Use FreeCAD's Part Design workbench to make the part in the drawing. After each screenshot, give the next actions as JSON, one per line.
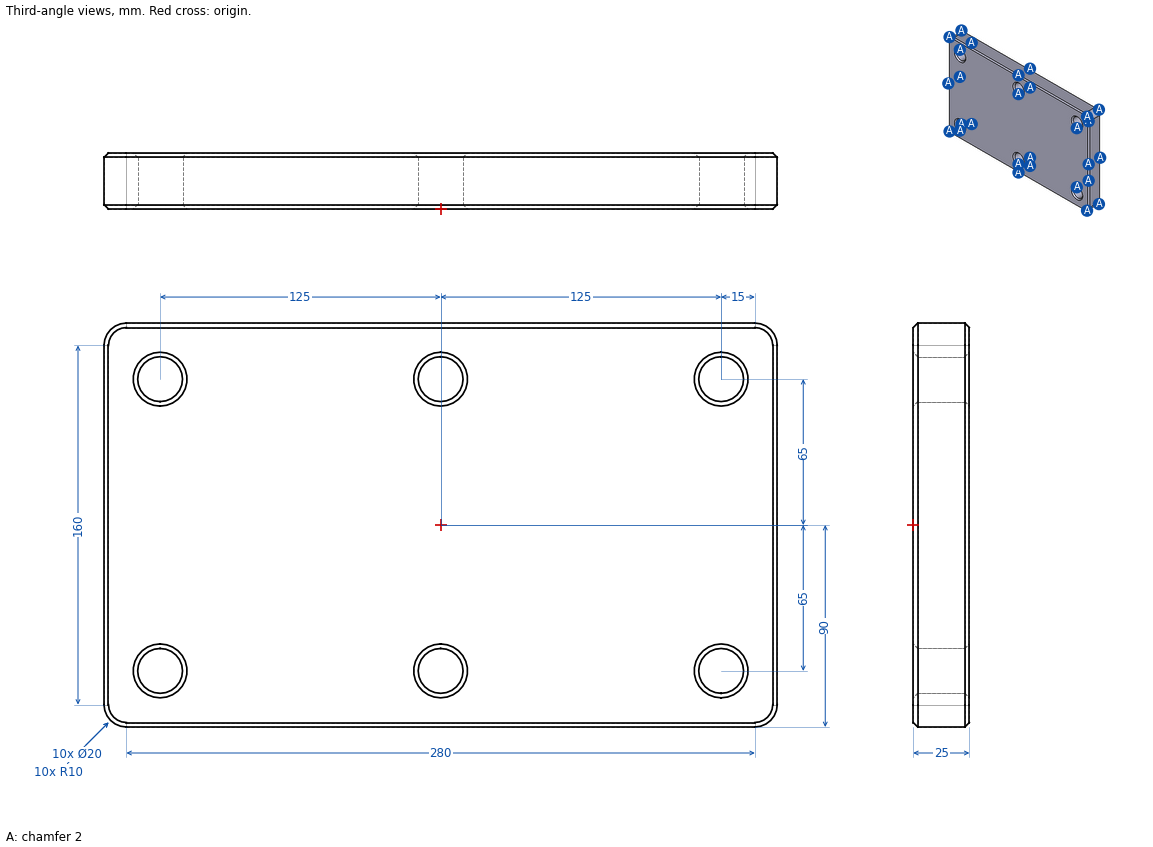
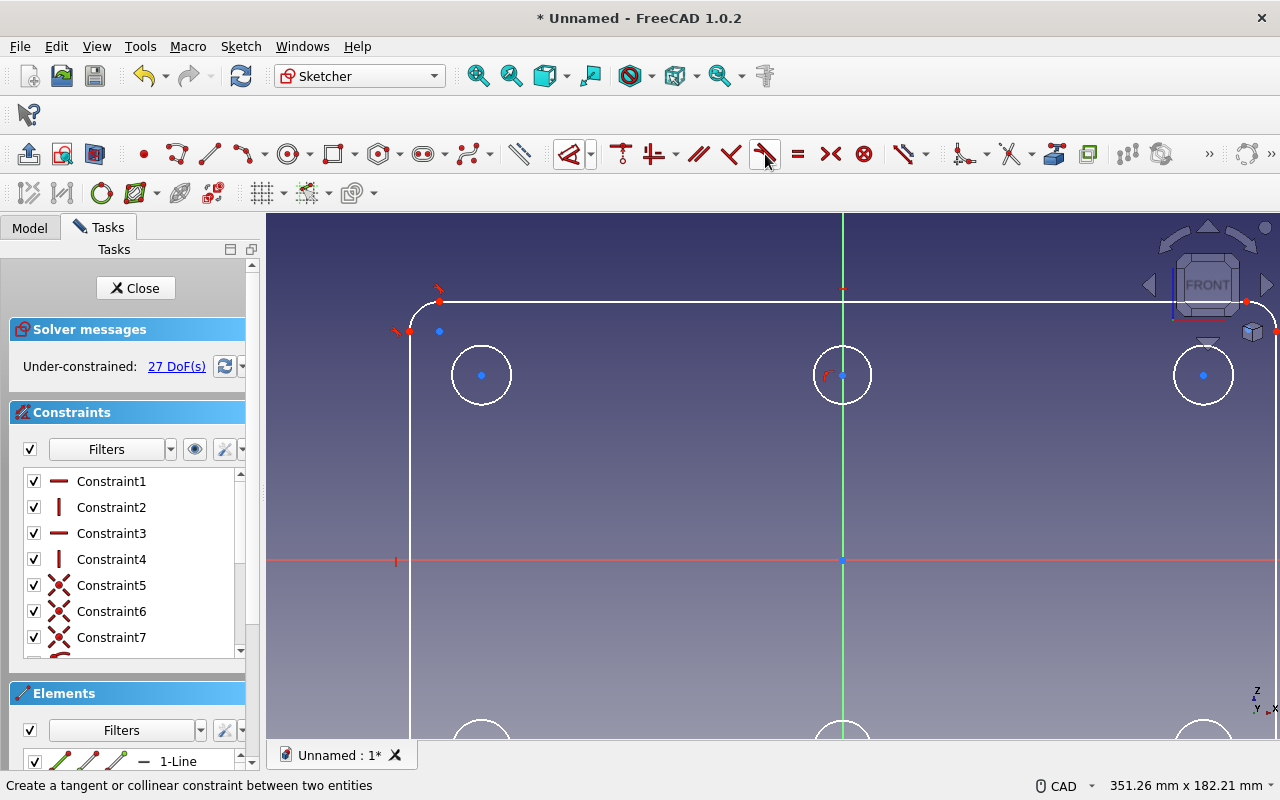
{"action": "left_click", "coordinate": [682, 302]}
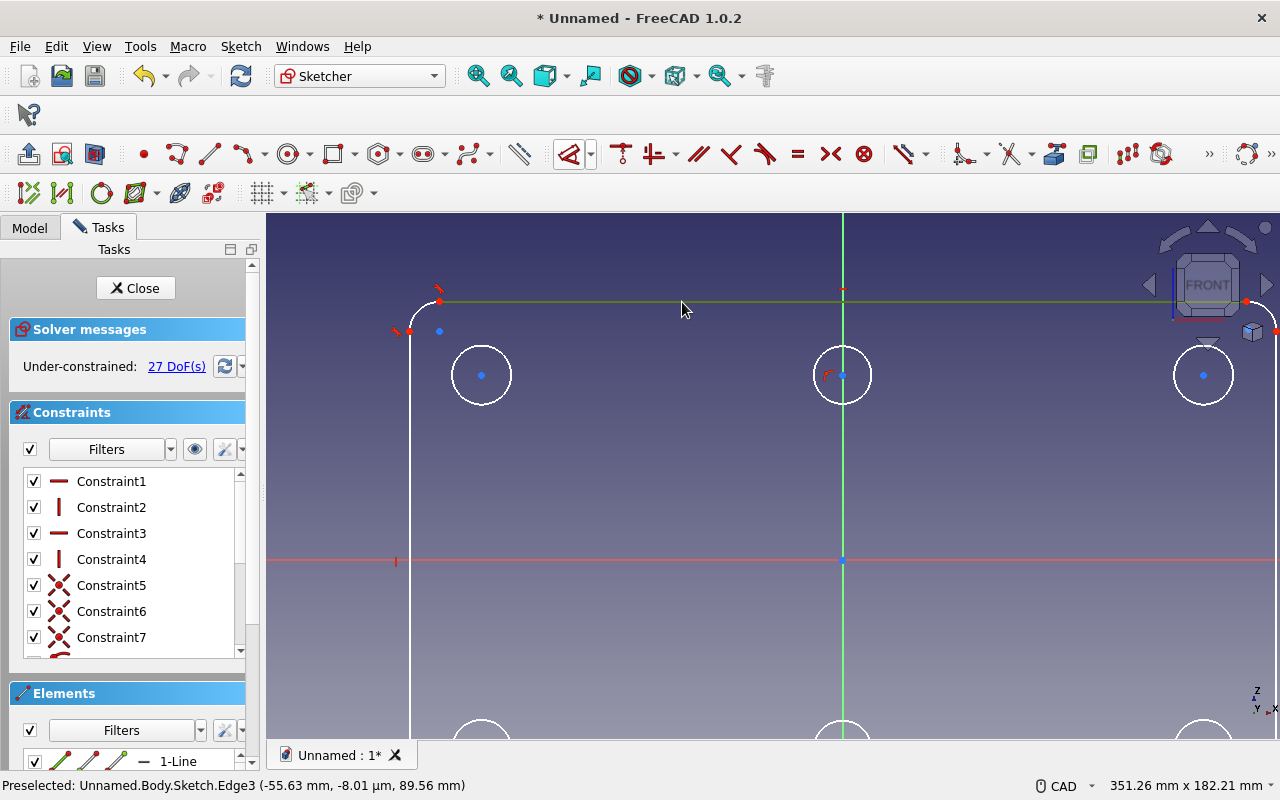
{"action": "scroll", "coordinate": [424, 304], "scroll_direction": "down", "scroll_amount": 2}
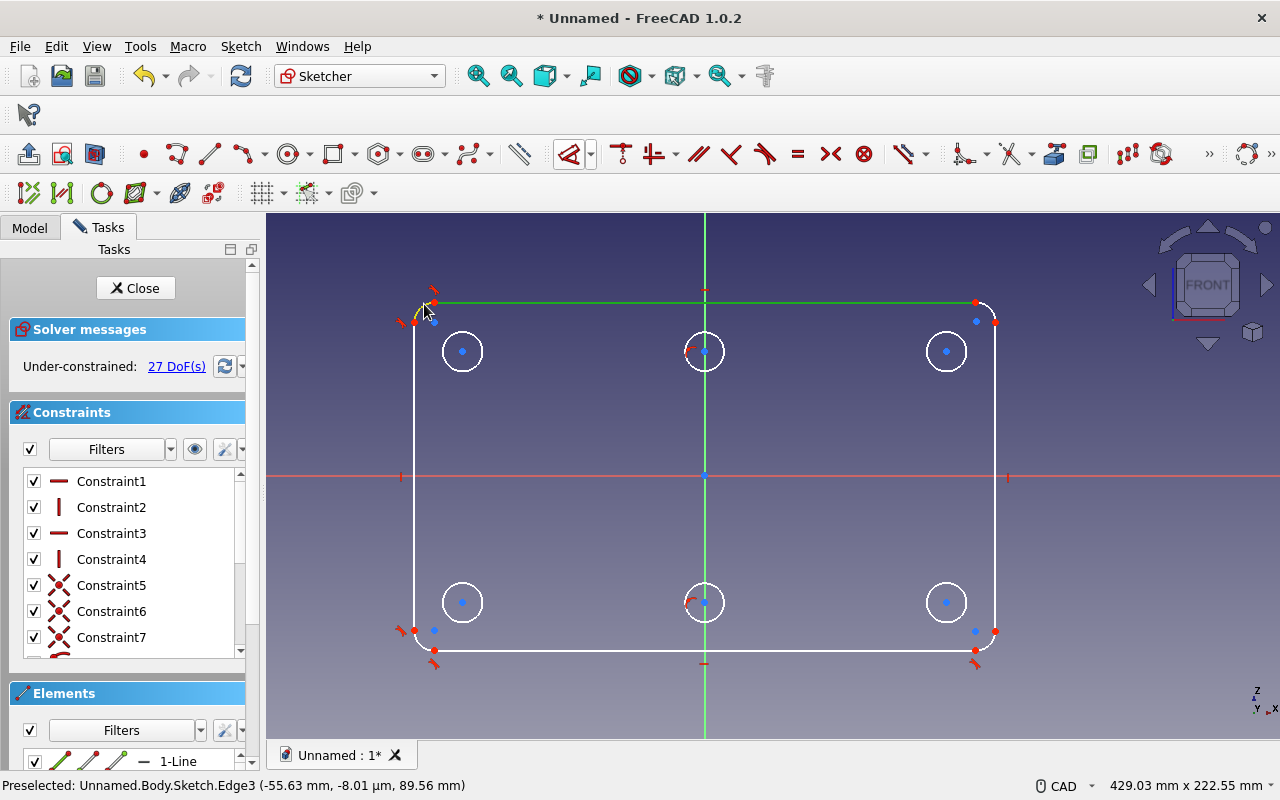
{"action": "scroll", "coordinate": [994, 313], "scroll_direction": "up", "scroll_amount": 2}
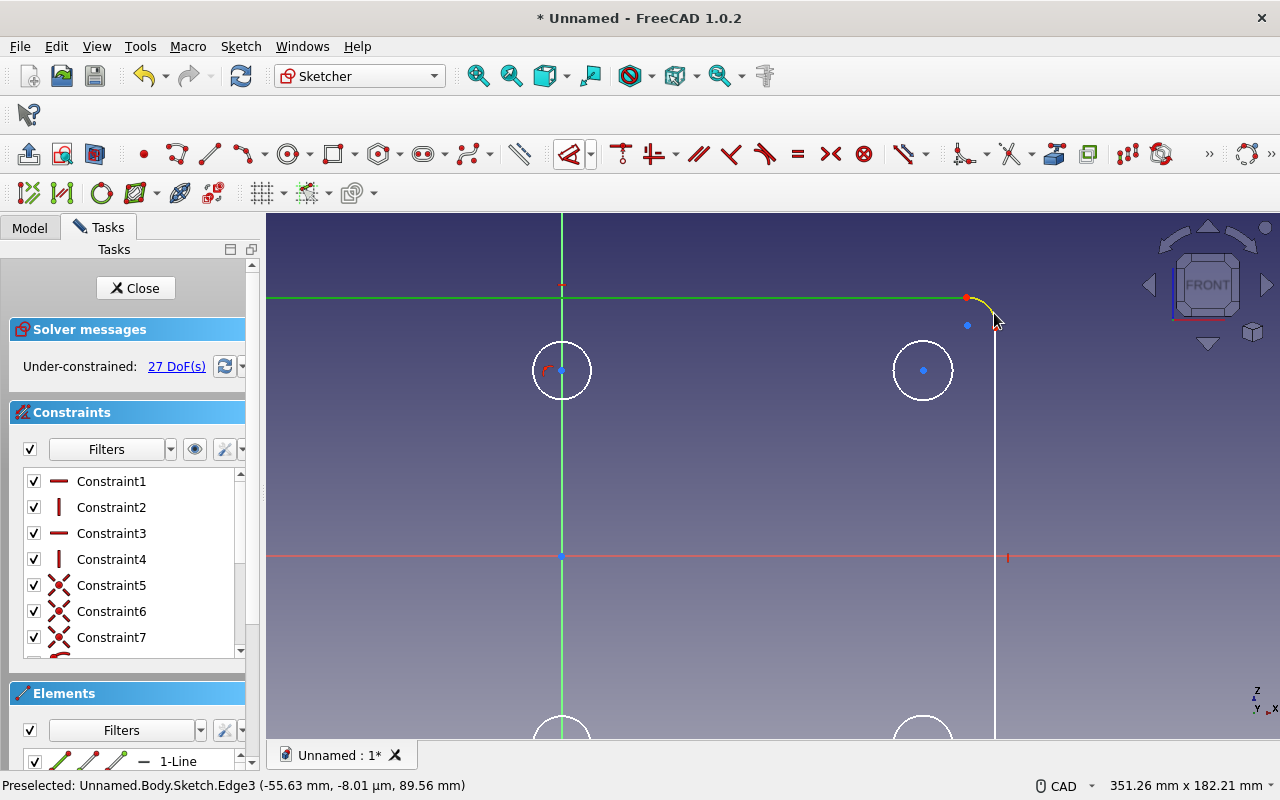
{"action": "left_click", "coordinate": [993, 314]}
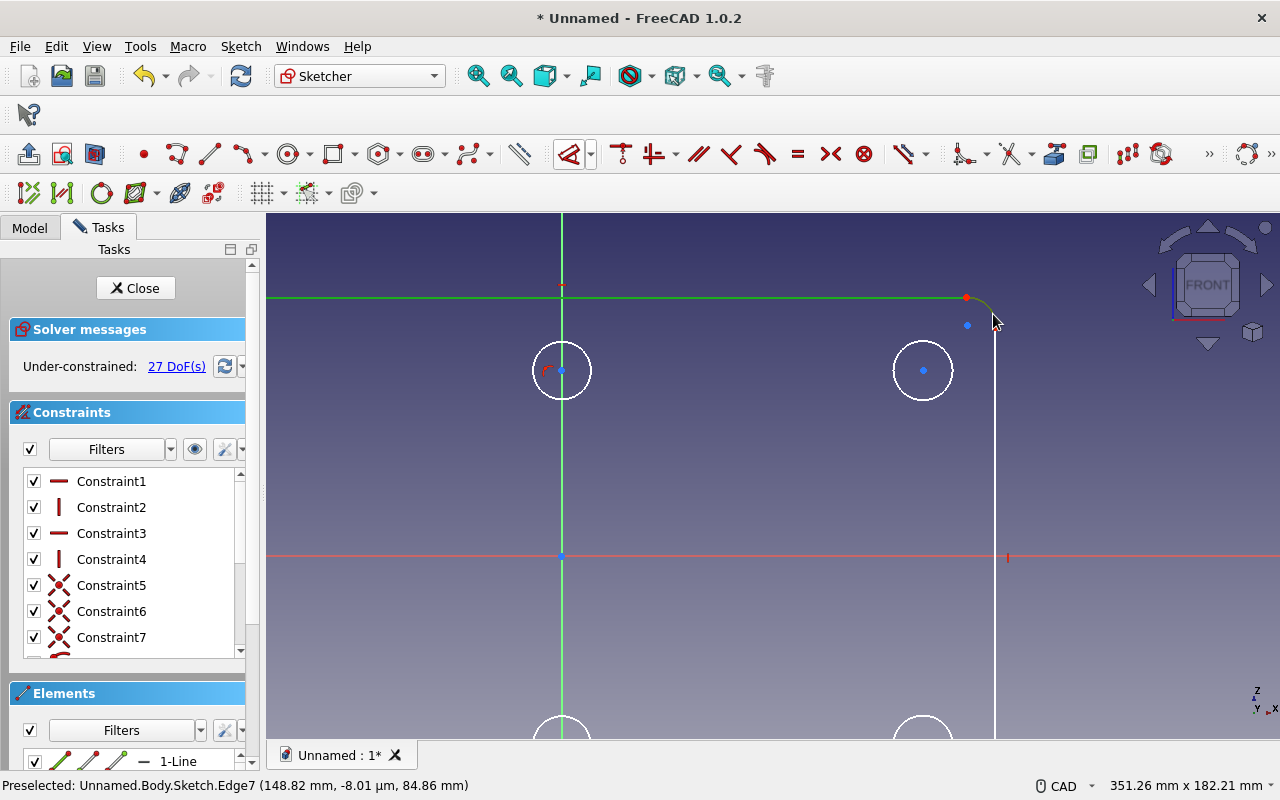
{"action": "left_click", "coordinate": [765, 154]}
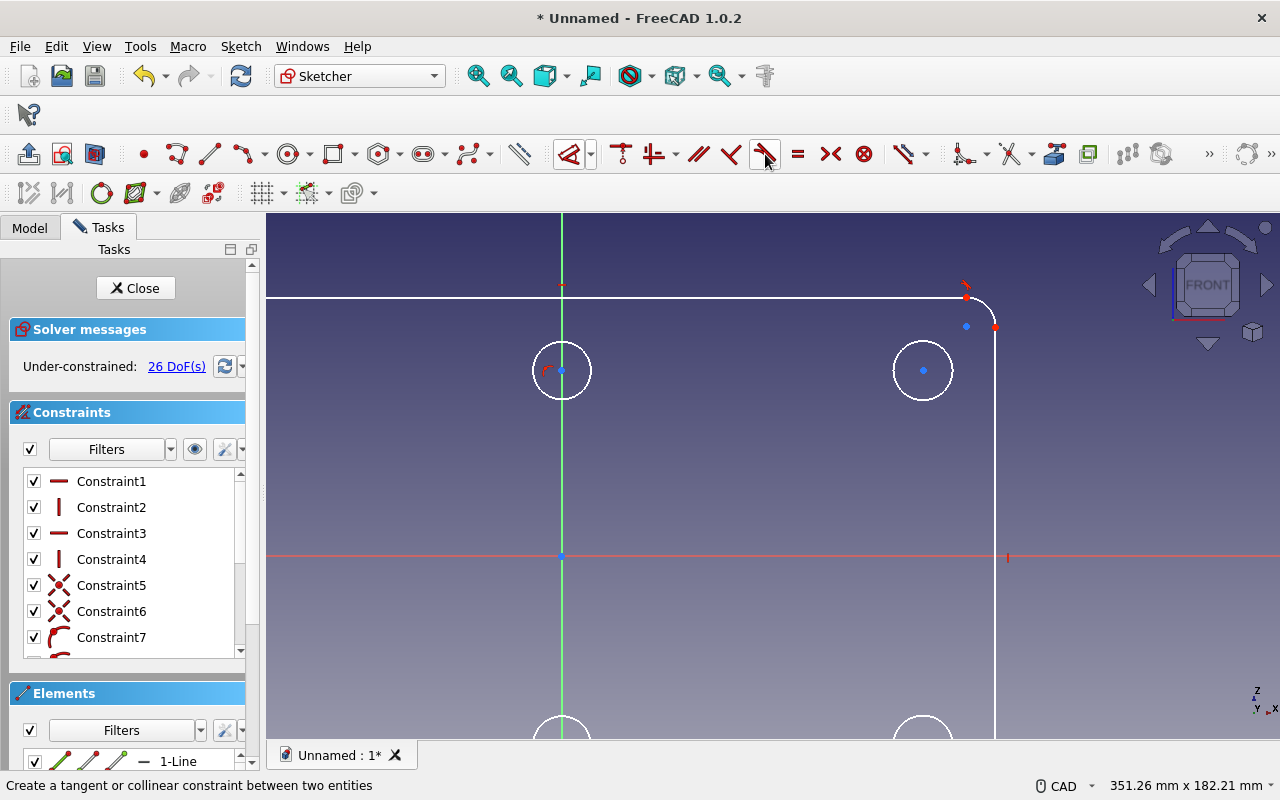
{"action": "left_click", "coordinate": [995, 466]}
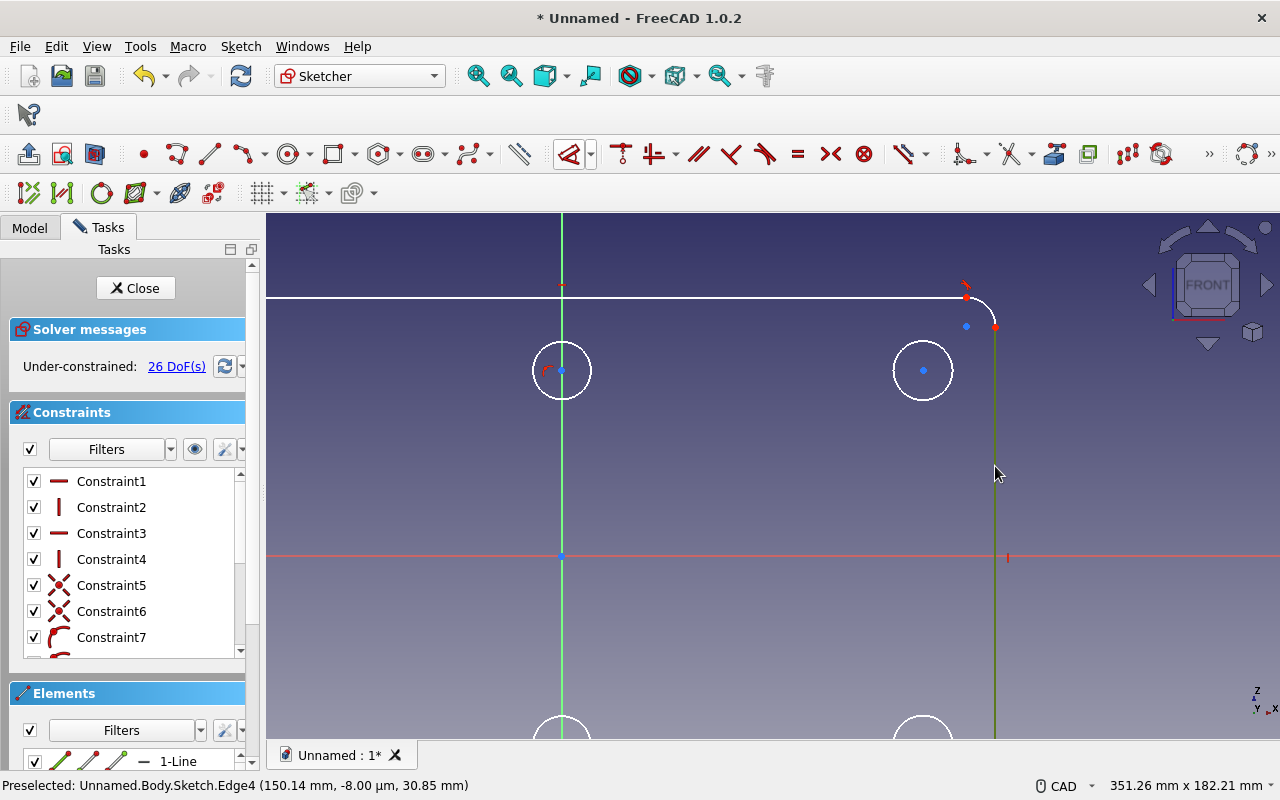
{"action": "left_click", "coordinate": [992, 314]}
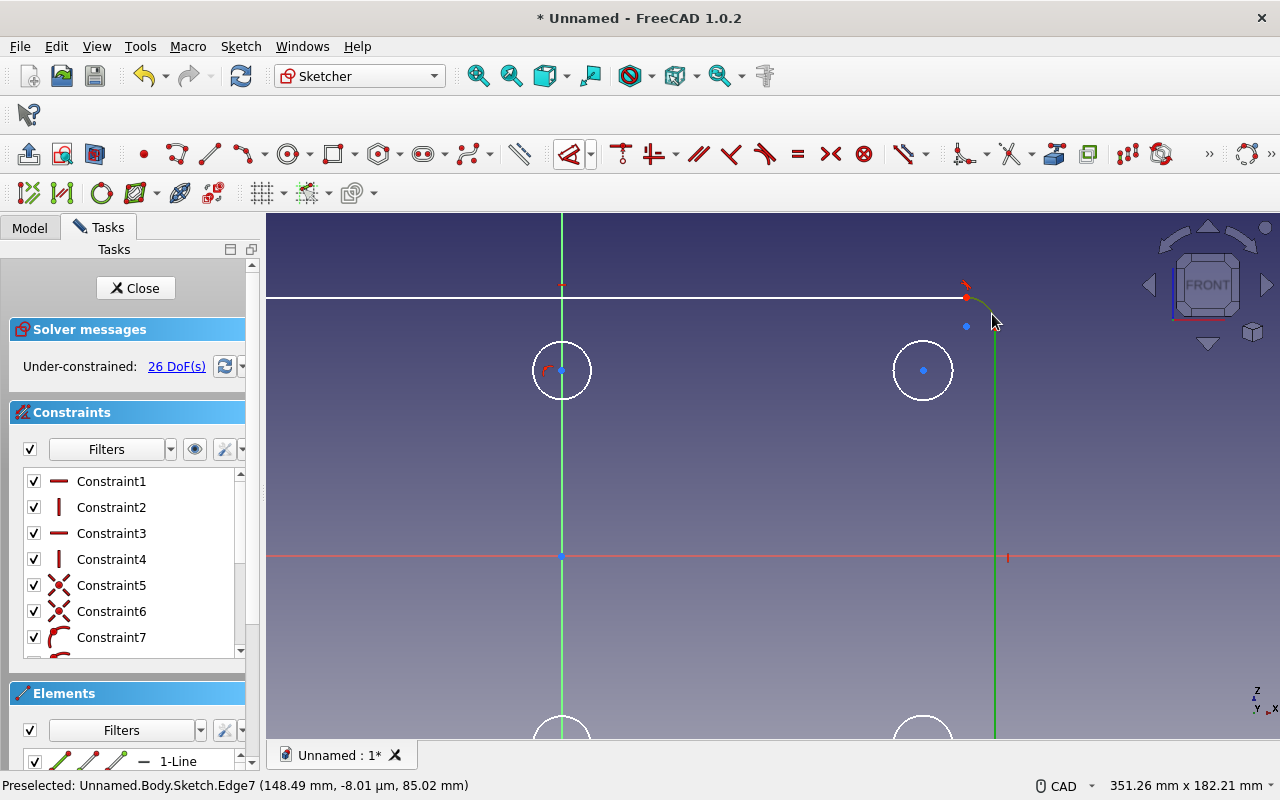
{"action": "left_click", "coordinate": [765, 154]}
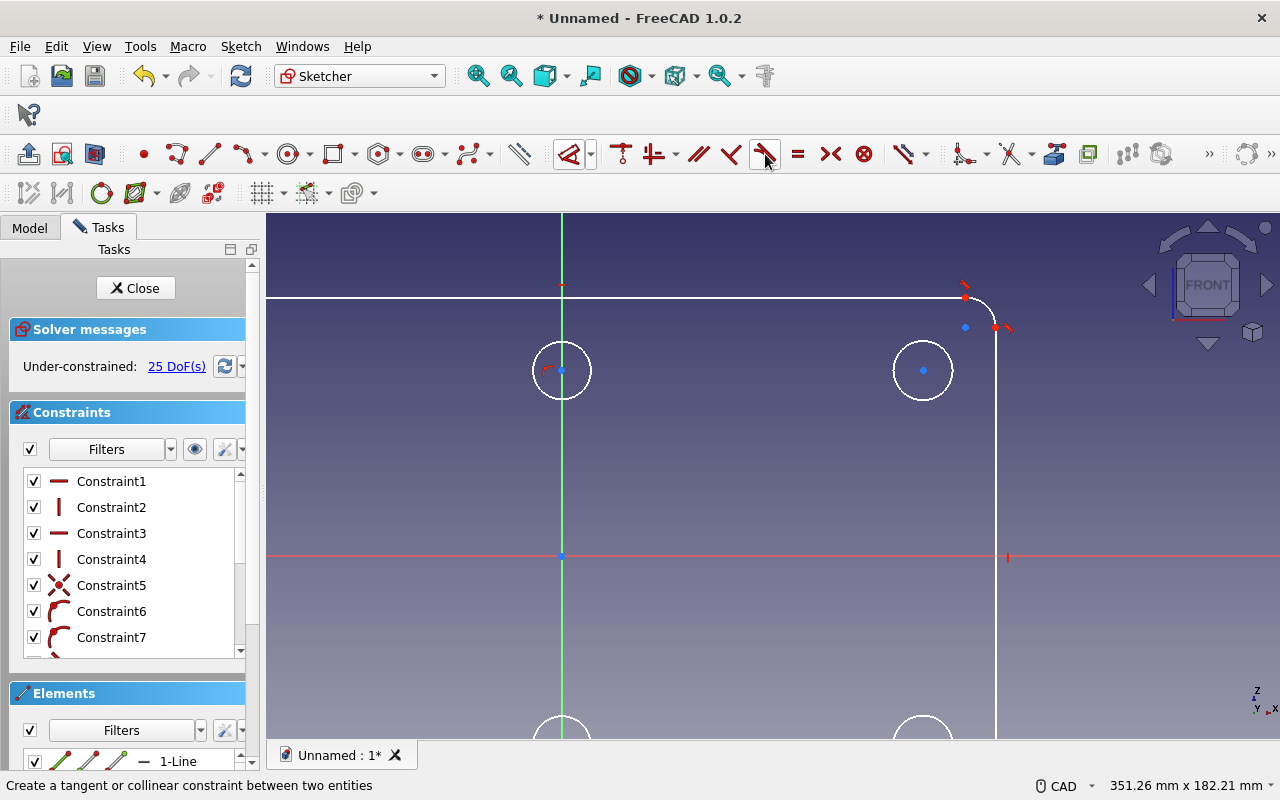
{"action": "left_click", "coordinate": [996, 466]}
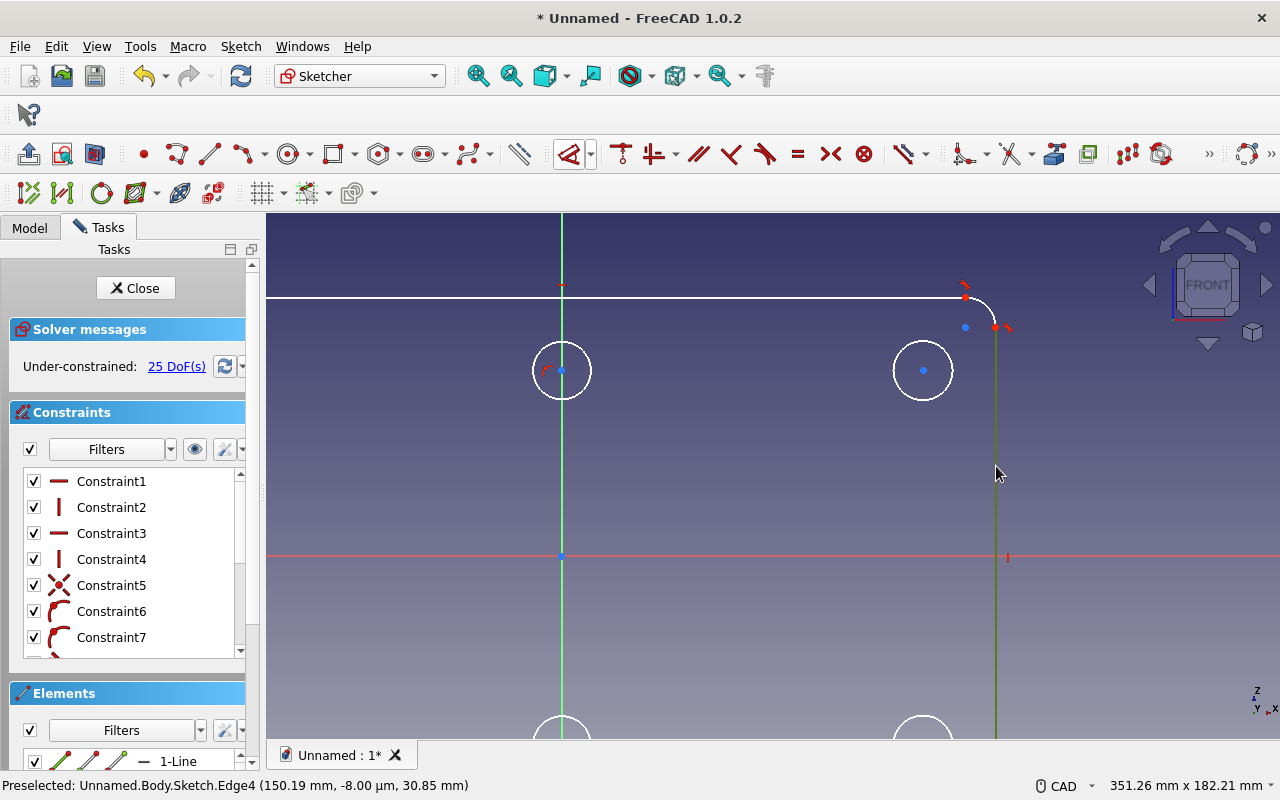
{"action": "scroll", "coordinate": [994, 313], "scroll_direction": "down", "scroll_amount": 2}